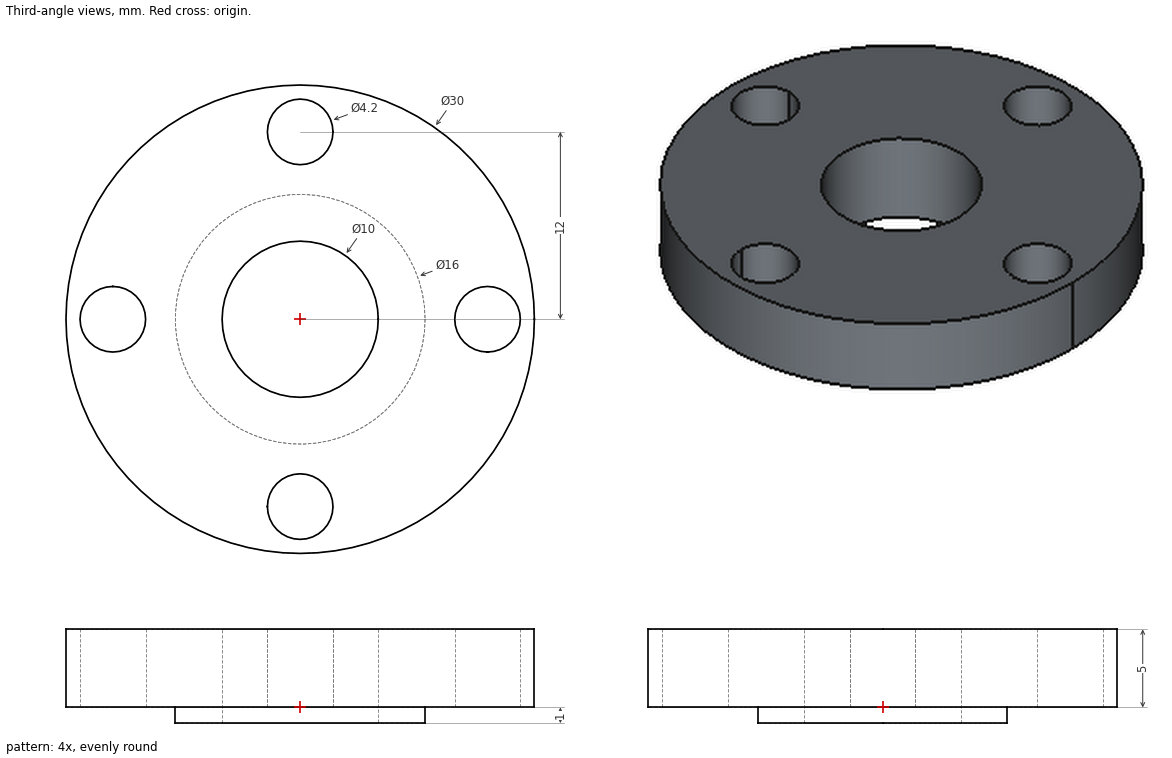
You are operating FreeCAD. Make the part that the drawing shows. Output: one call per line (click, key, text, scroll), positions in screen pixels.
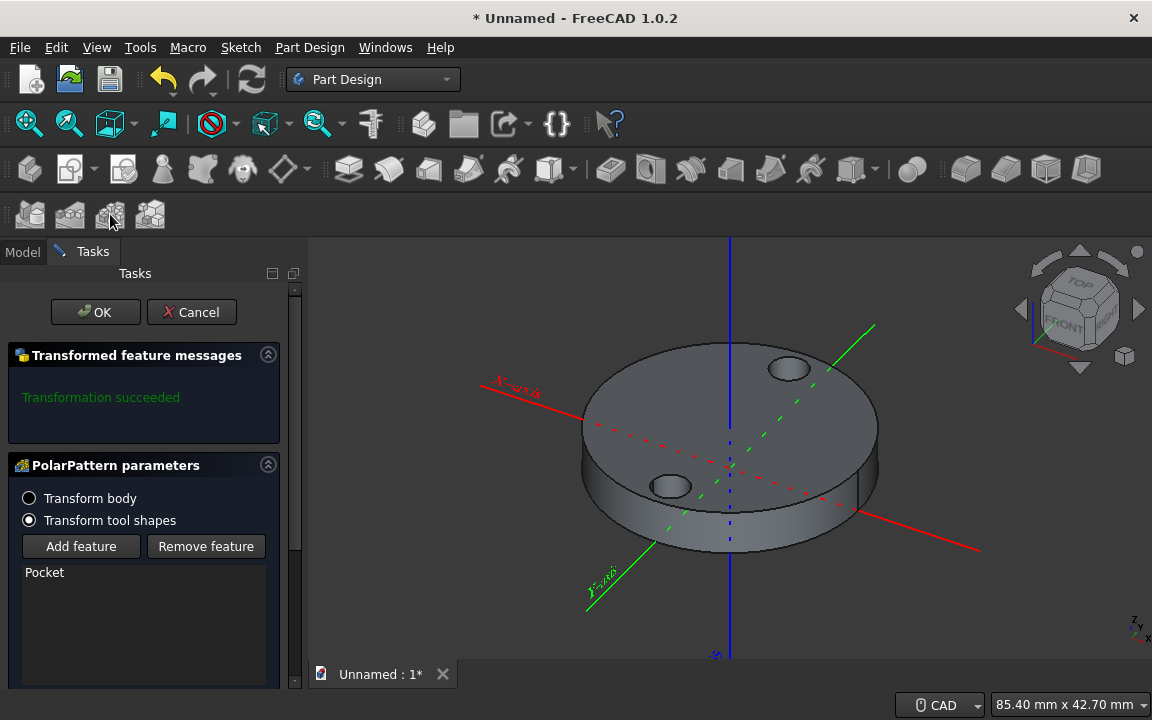
scroll(295, 486, down, 2)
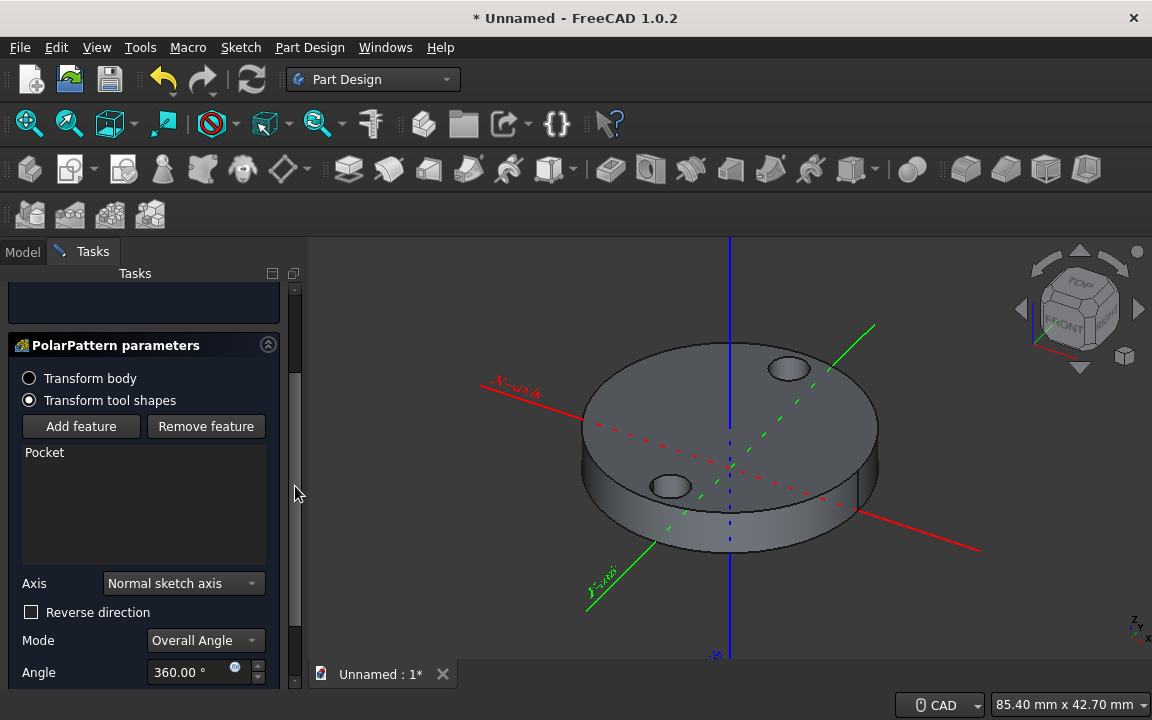
click(184, 584)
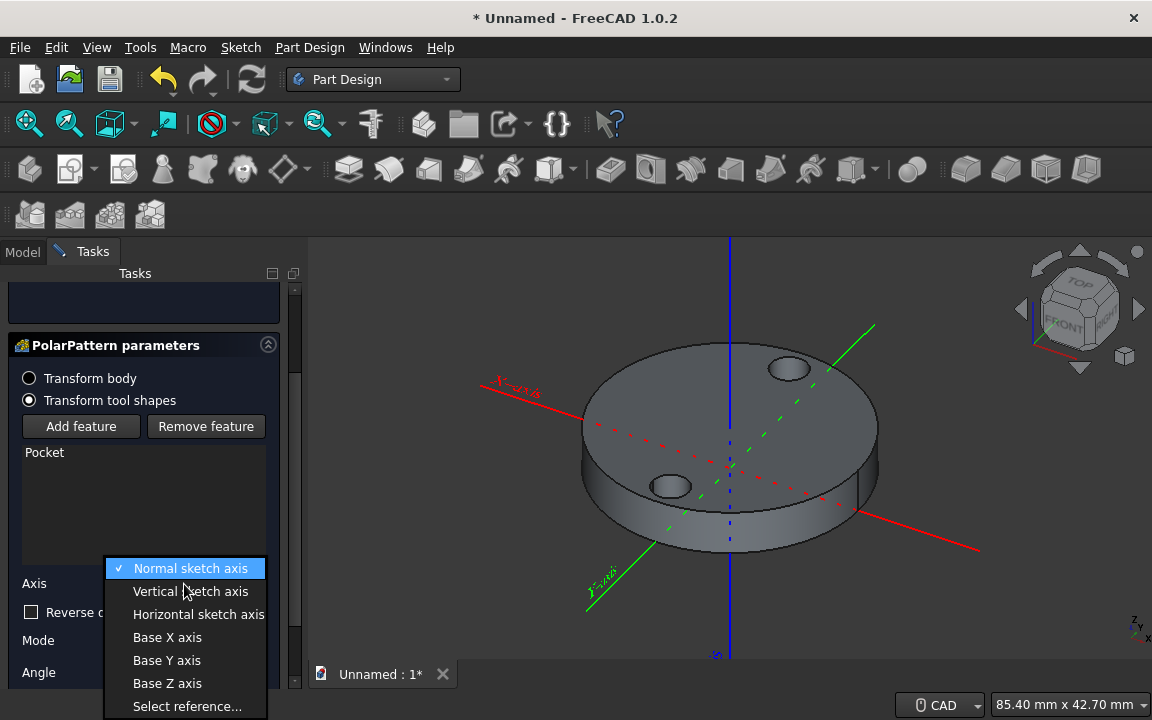
click(184, 684)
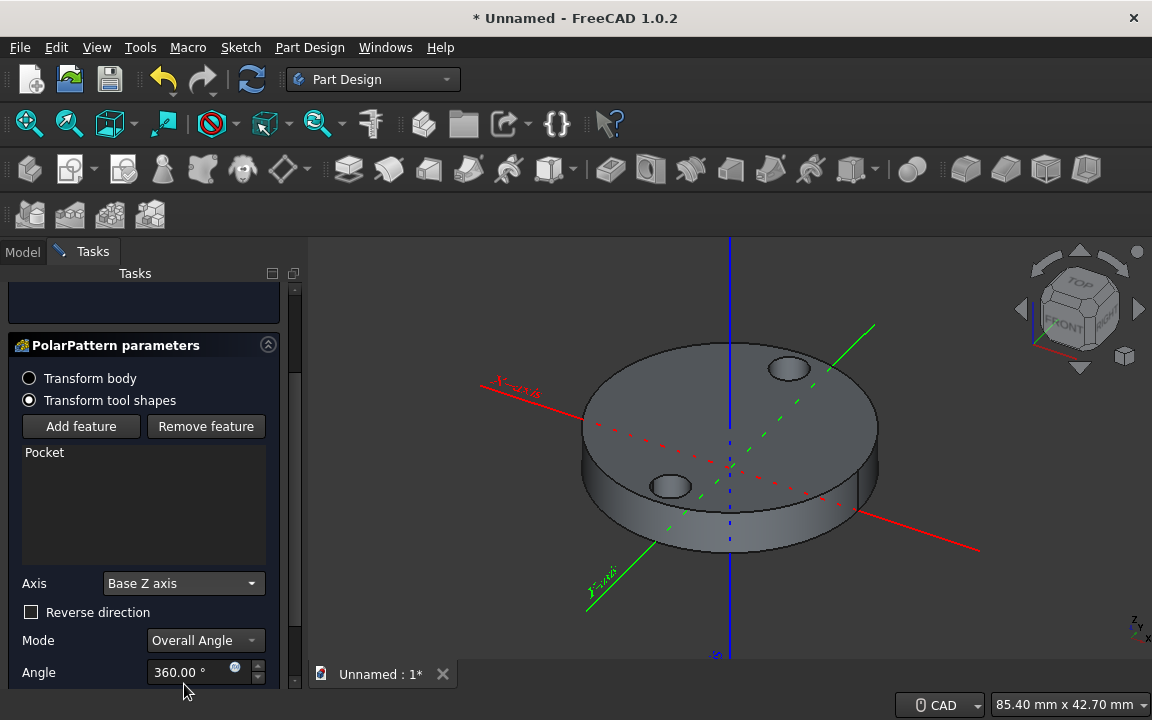
scroll(295, 486, down, 2)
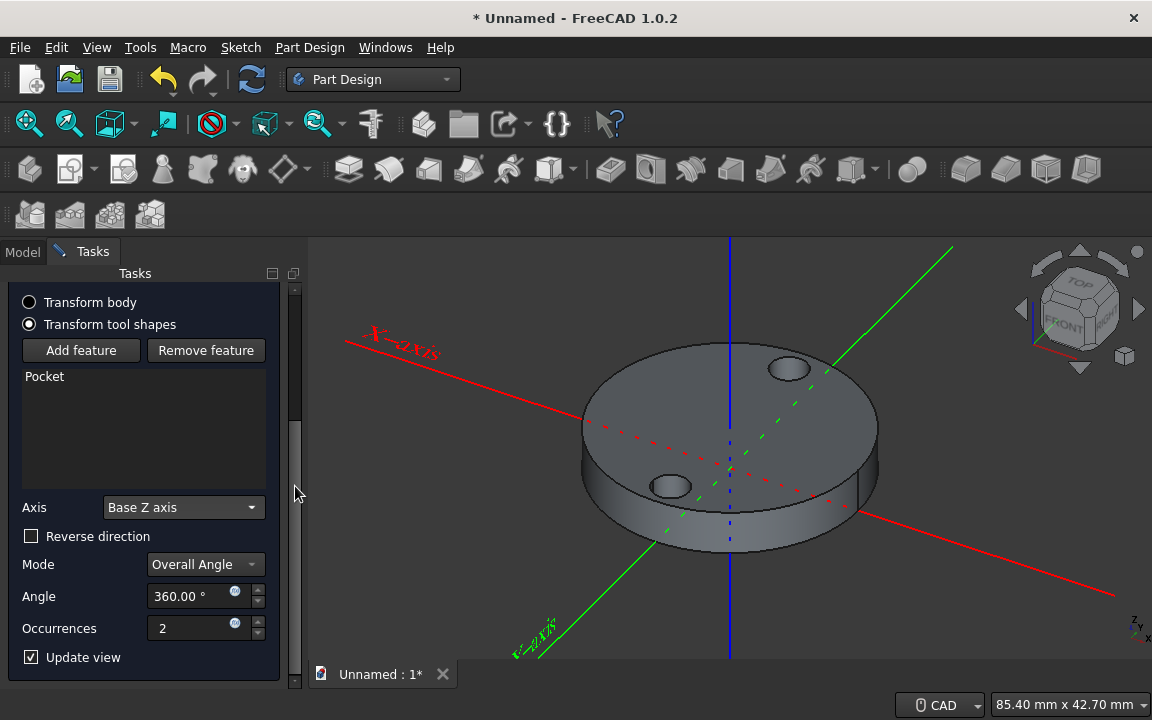
triple_click(198, 628)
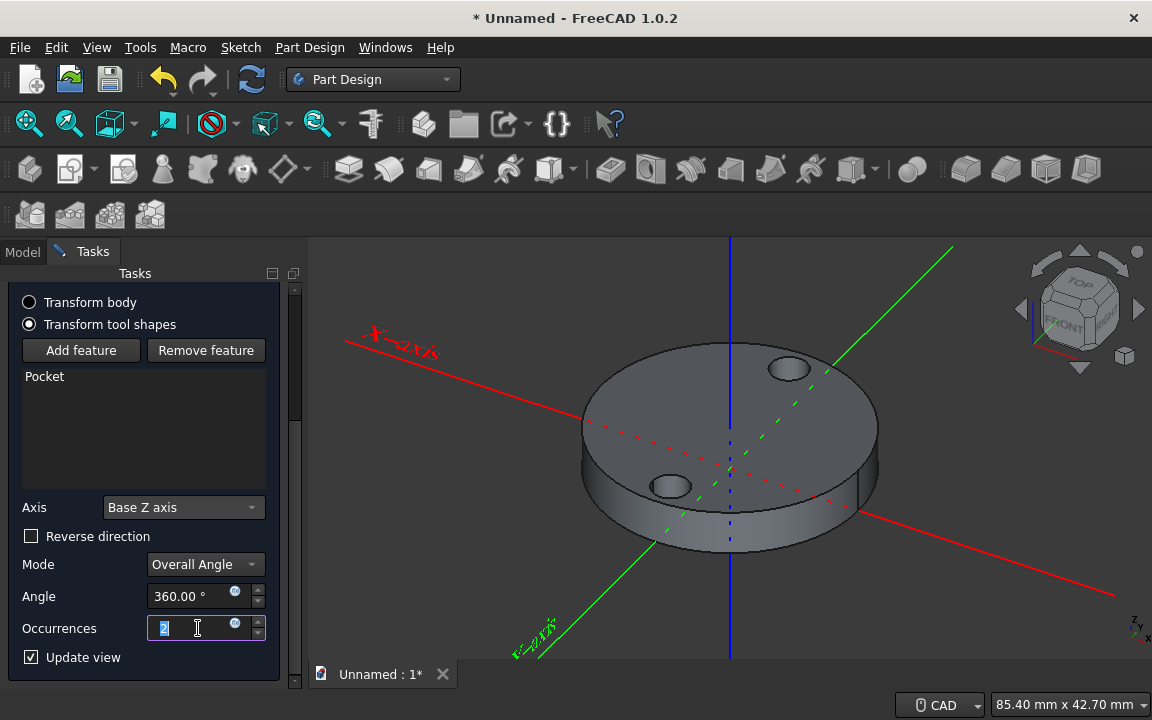
text(4)
key(Tab)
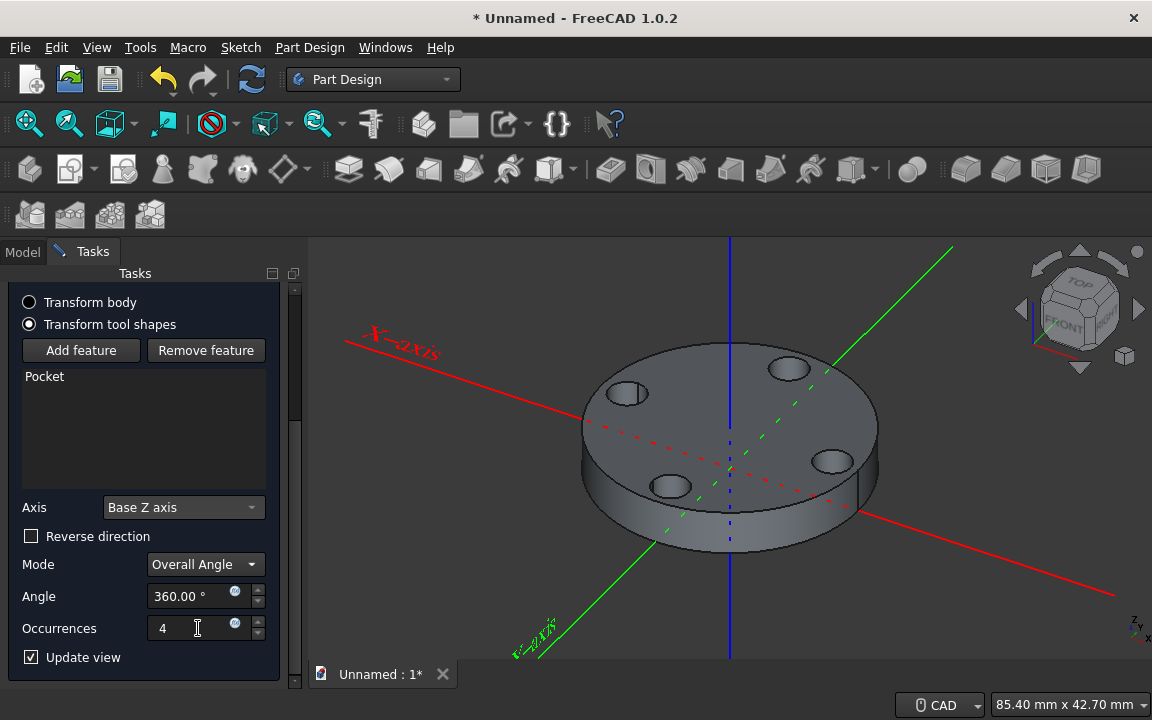
scroll(295, 486, up, 5)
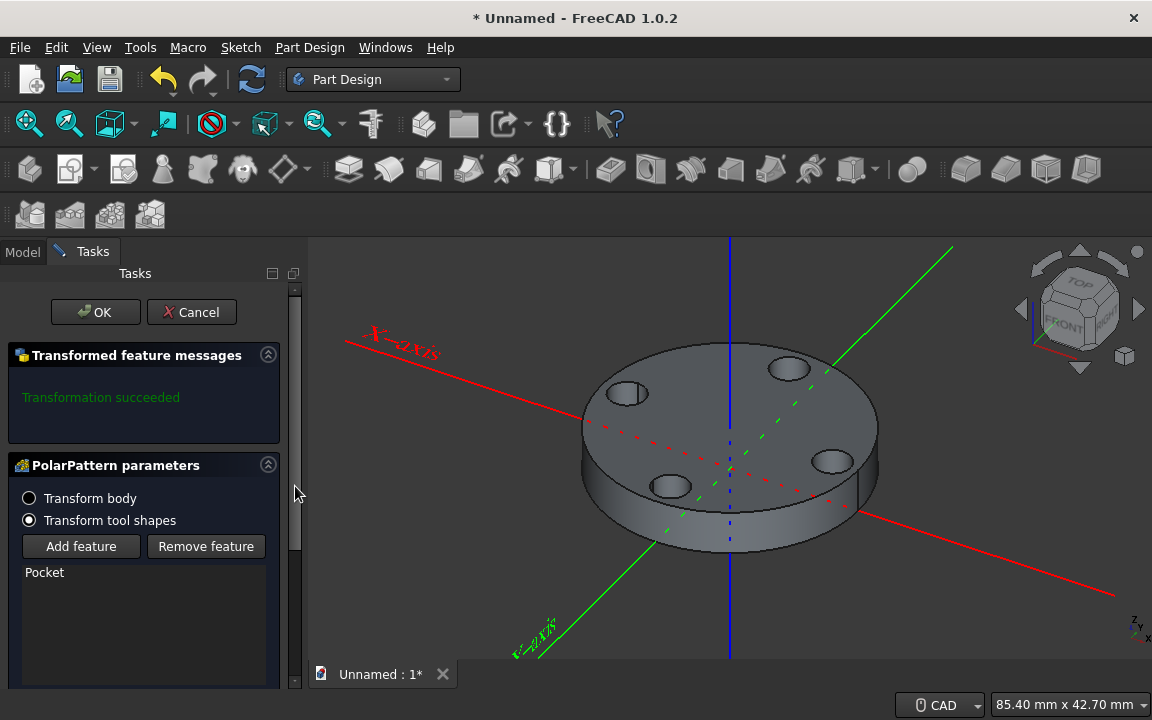
click(96, 312)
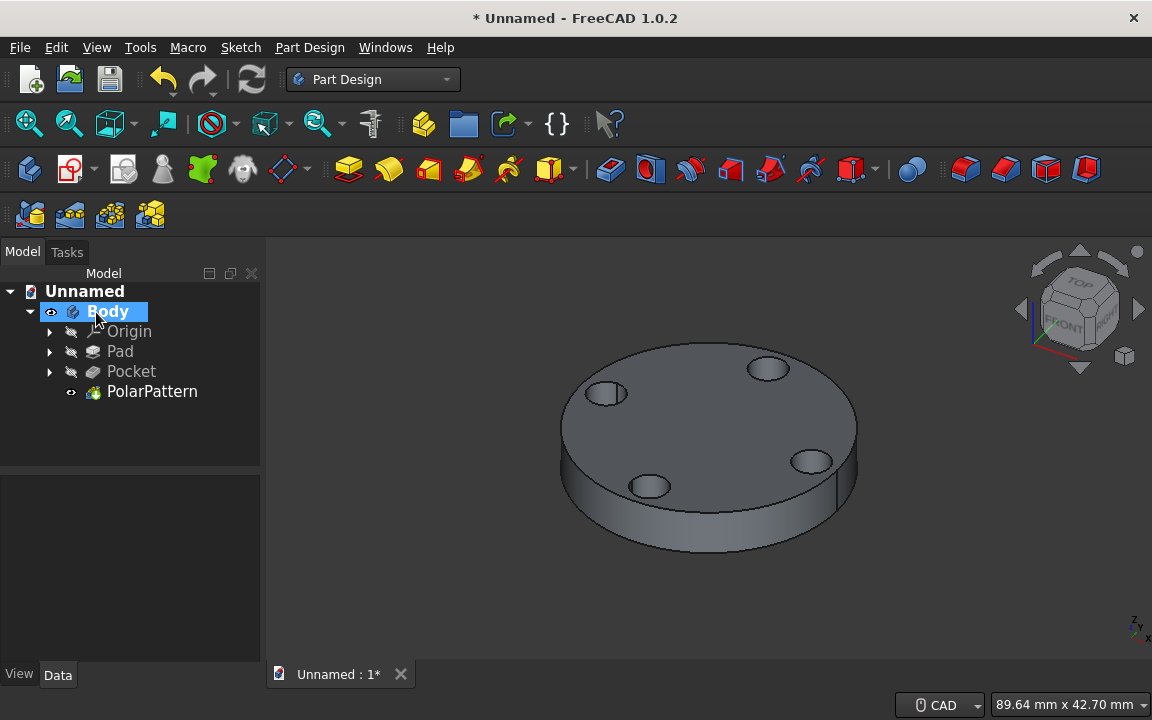
key(5)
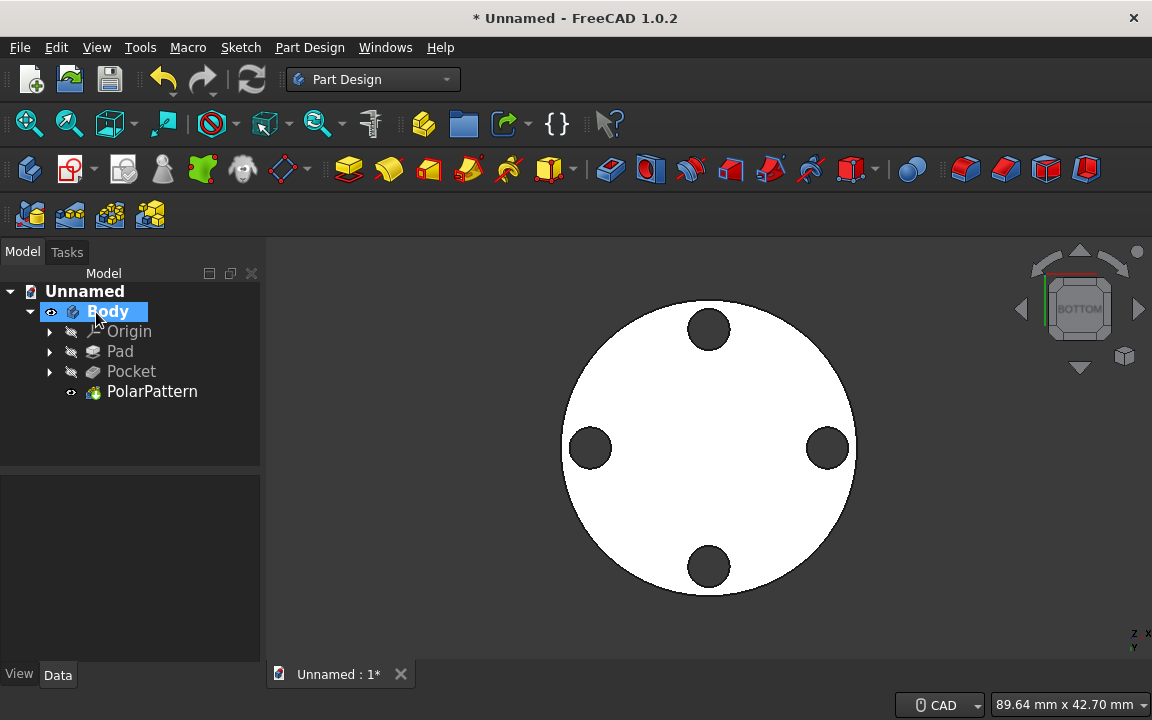
click(709, 447)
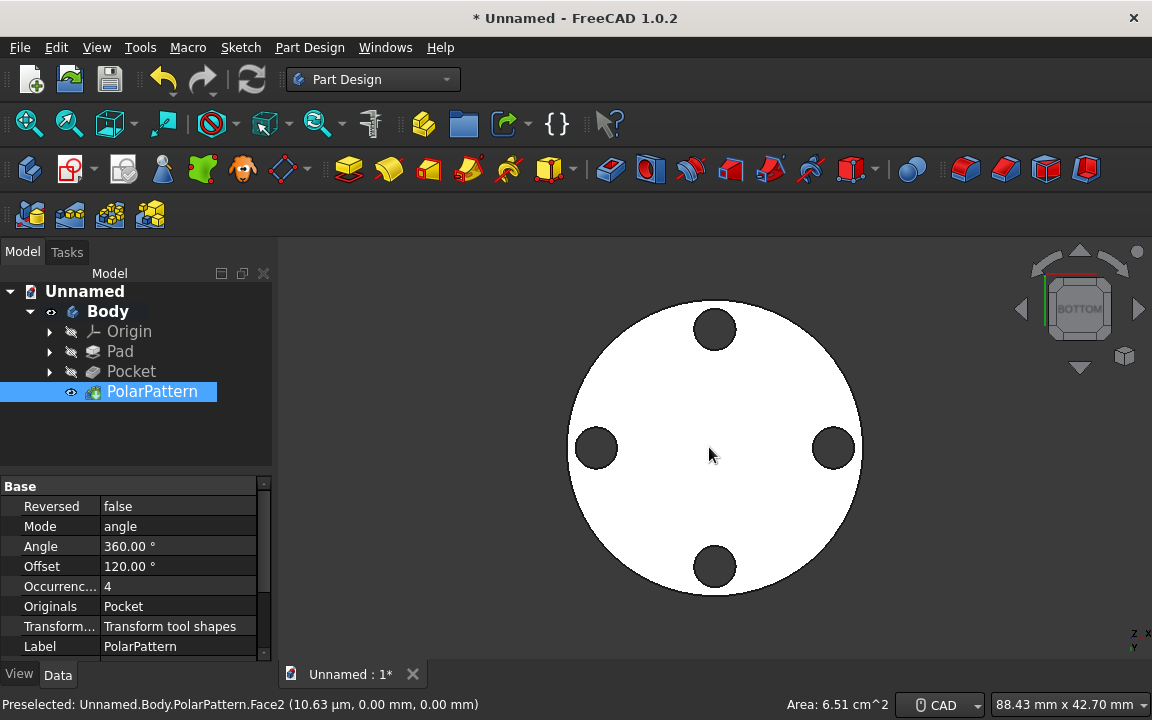
click(70, 170)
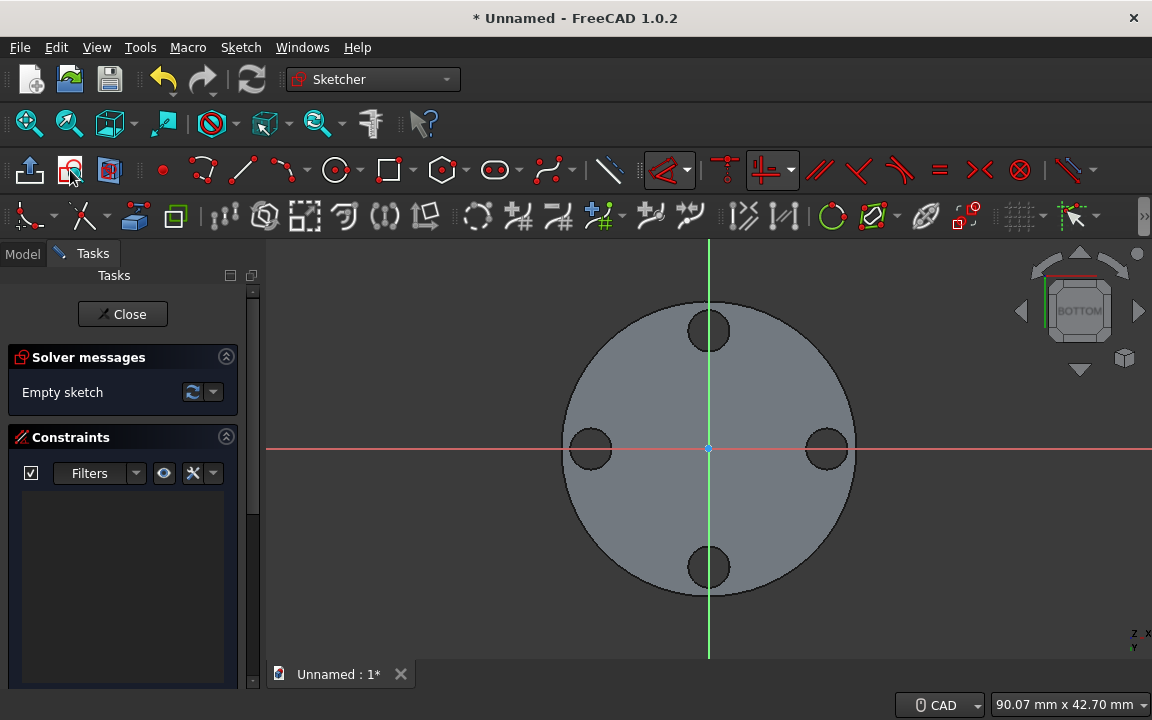
scroll(848, 449, up, 2)